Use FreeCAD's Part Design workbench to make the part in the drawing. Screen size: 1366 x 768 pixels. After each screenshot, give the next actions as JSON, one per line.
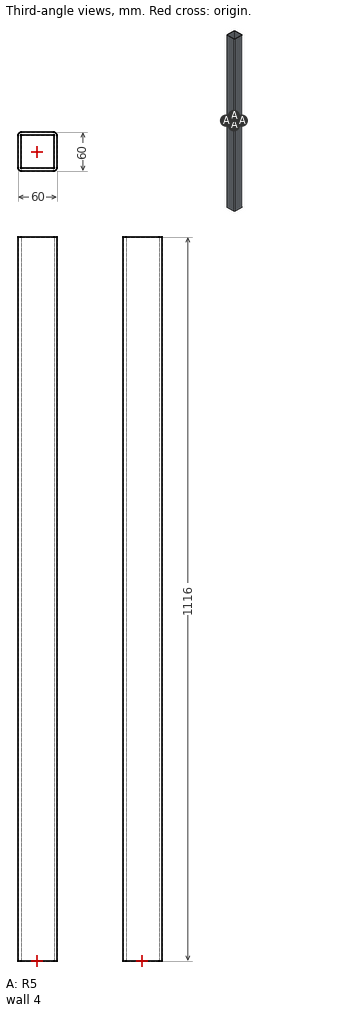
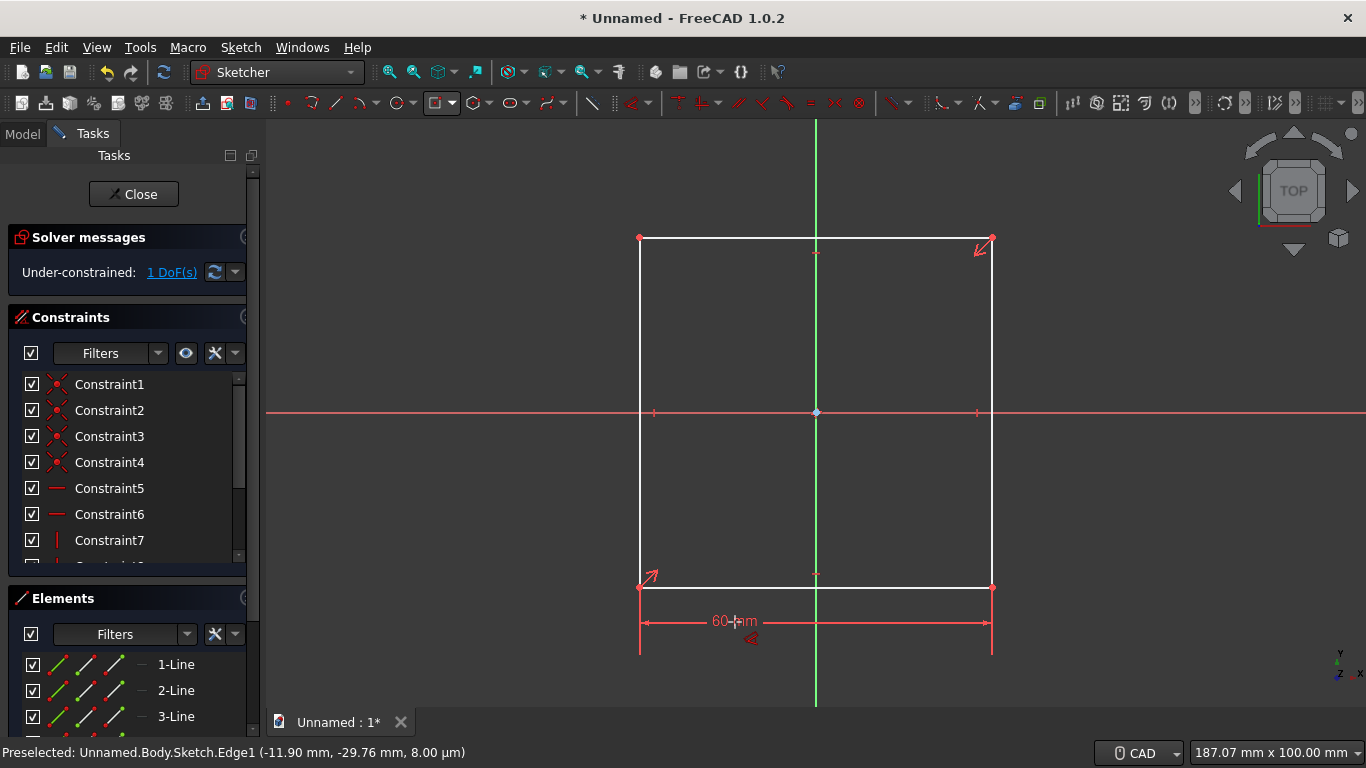
{"action": "left_click", "coordinate": [992, 483]}
{"action": "left_click", "coordinate": [1026, 333]}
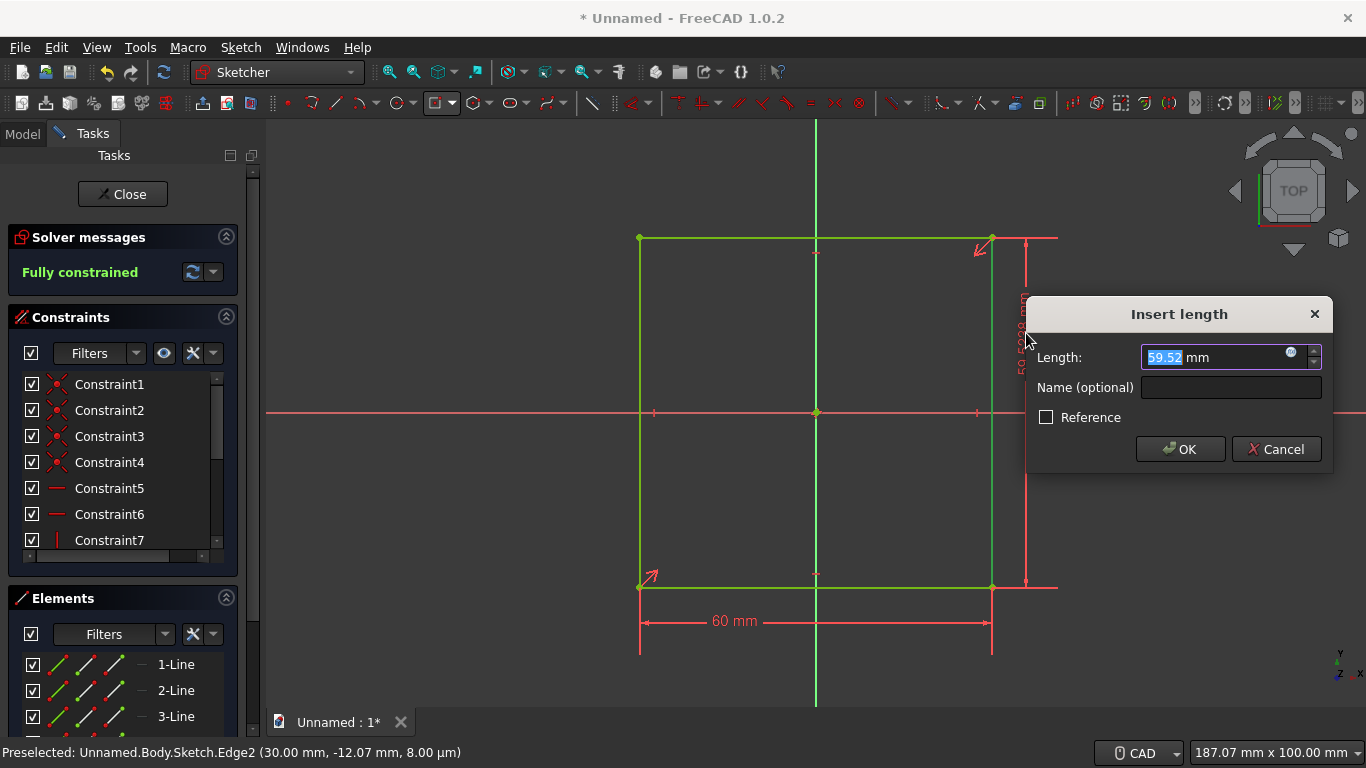
{"action": "type", "text": "60"}
{"action": "key", "text": "Return"}
{"action": "key", "text": "Escape"}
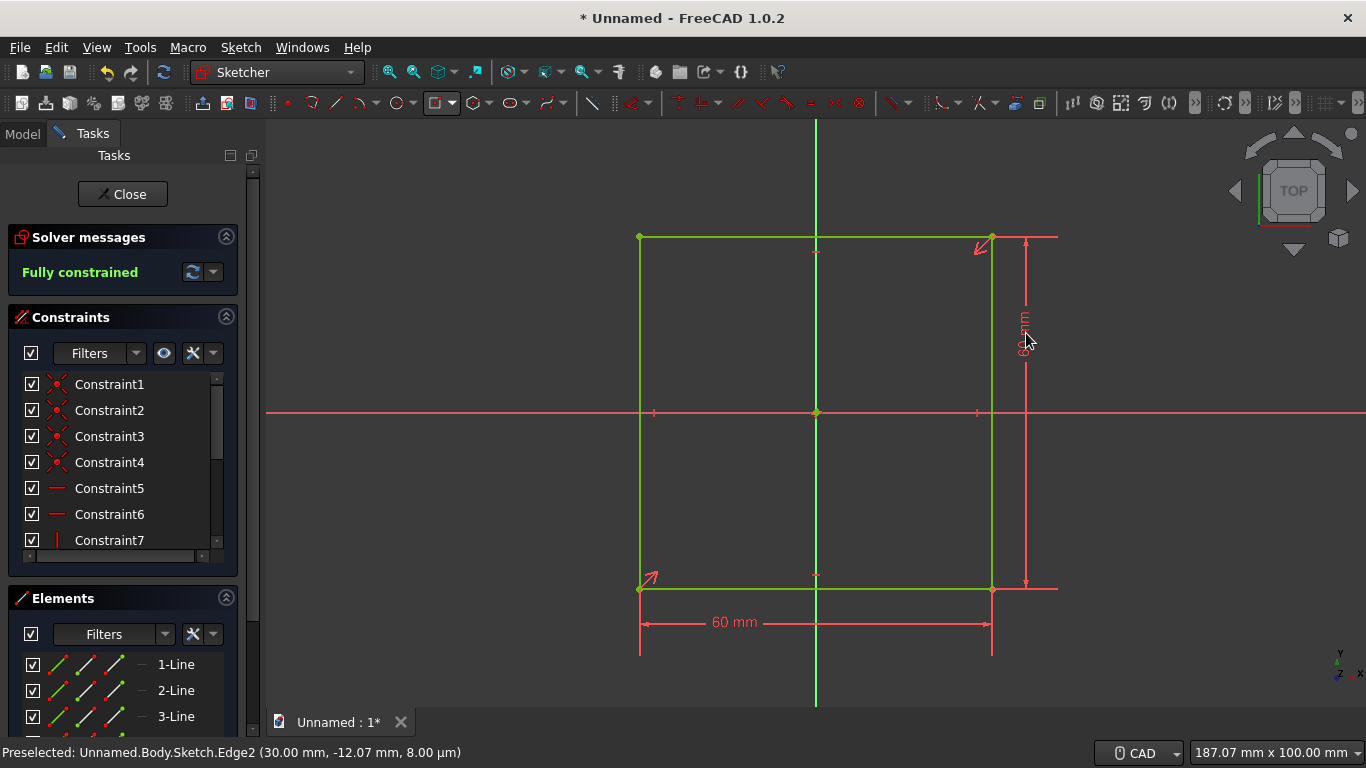
{"action": "left_click", "coordinate": [123, 194]}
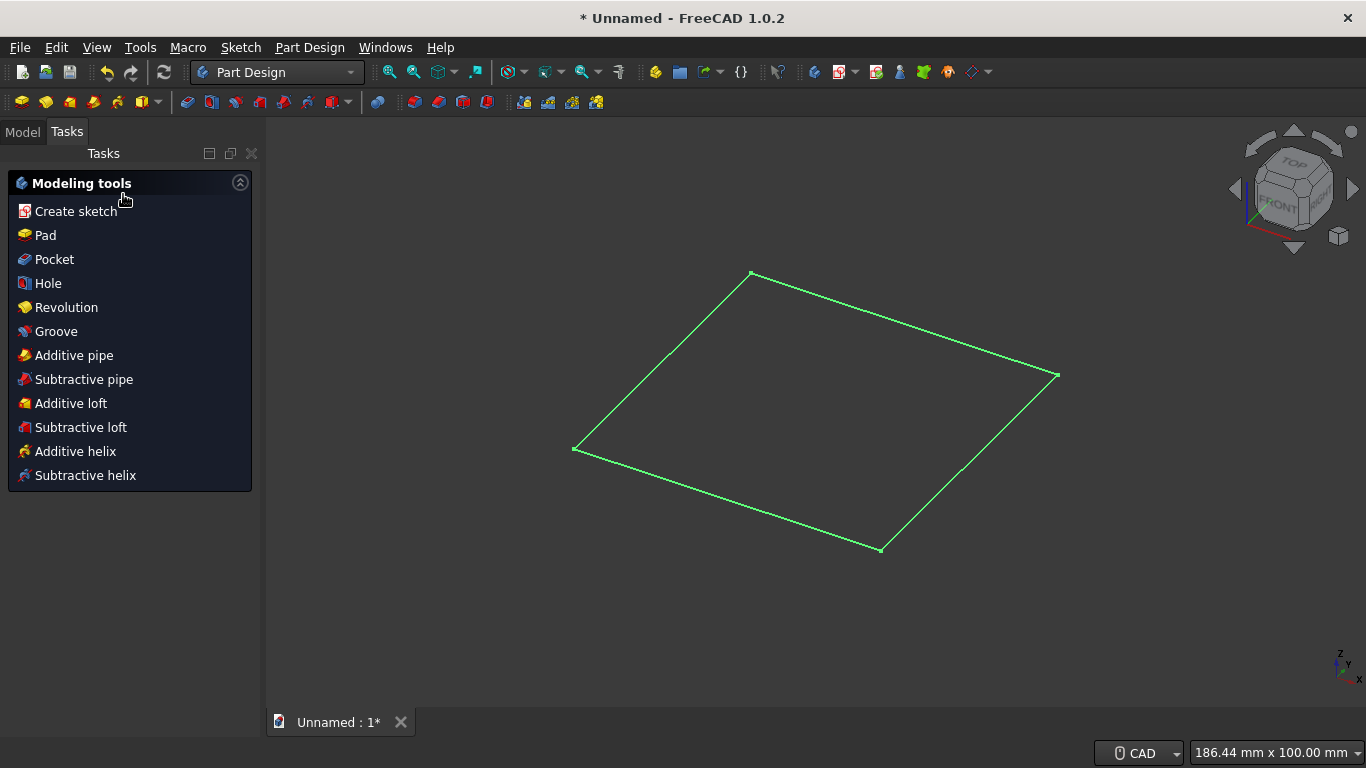
{"action": "left_click", "coordinate": [22, 102]}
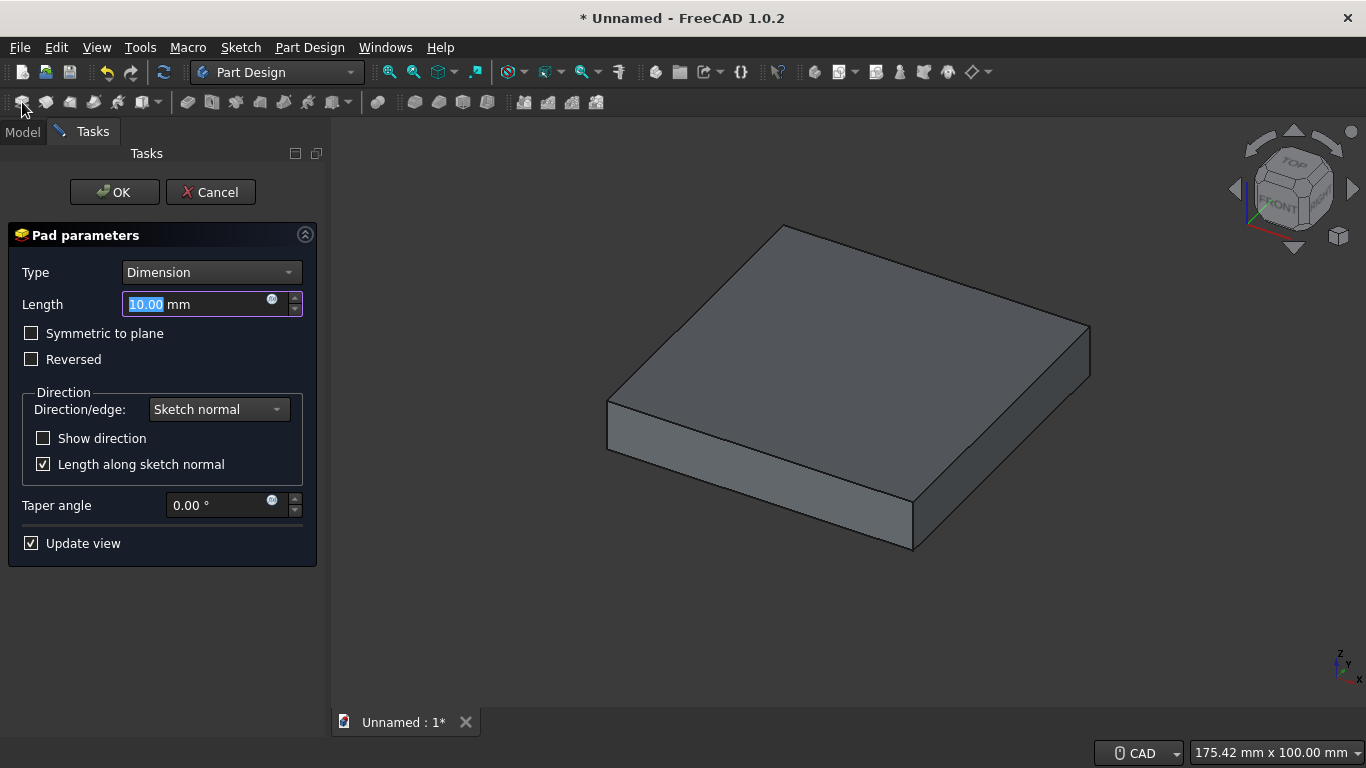
{"action": "type", "text": "1116"}
{"action": "key", "text": "Tab"}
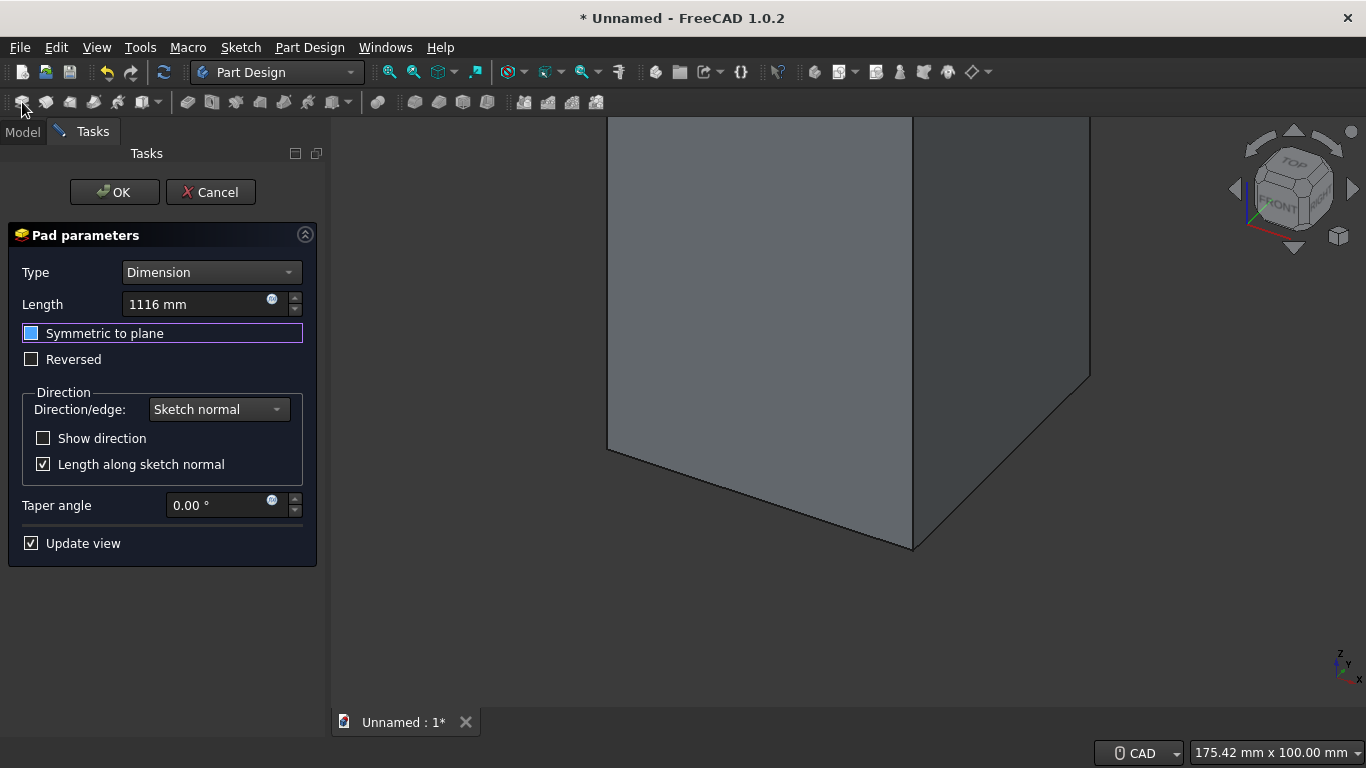
{"action": "left_click", "coordinate": [115, 192]}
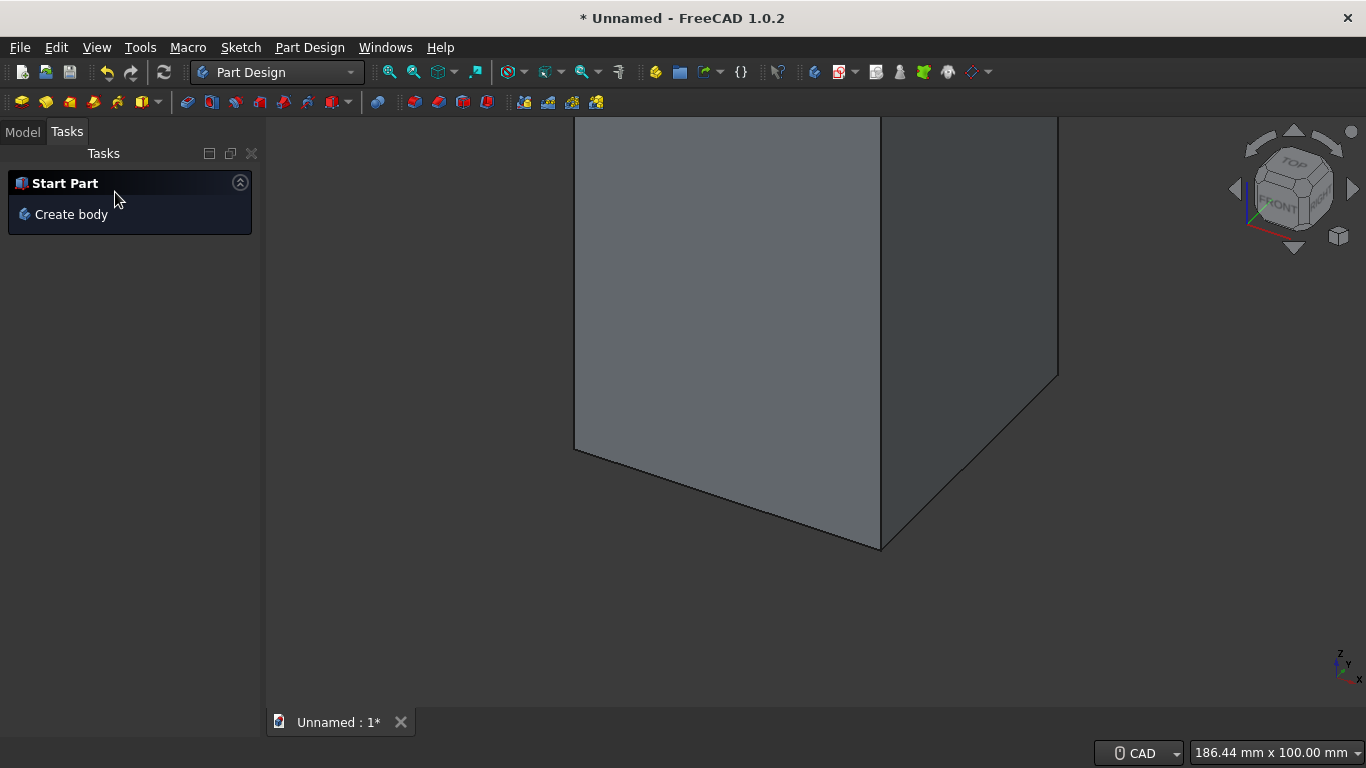
{"action": "left_click", "coordinate": [390, 72]}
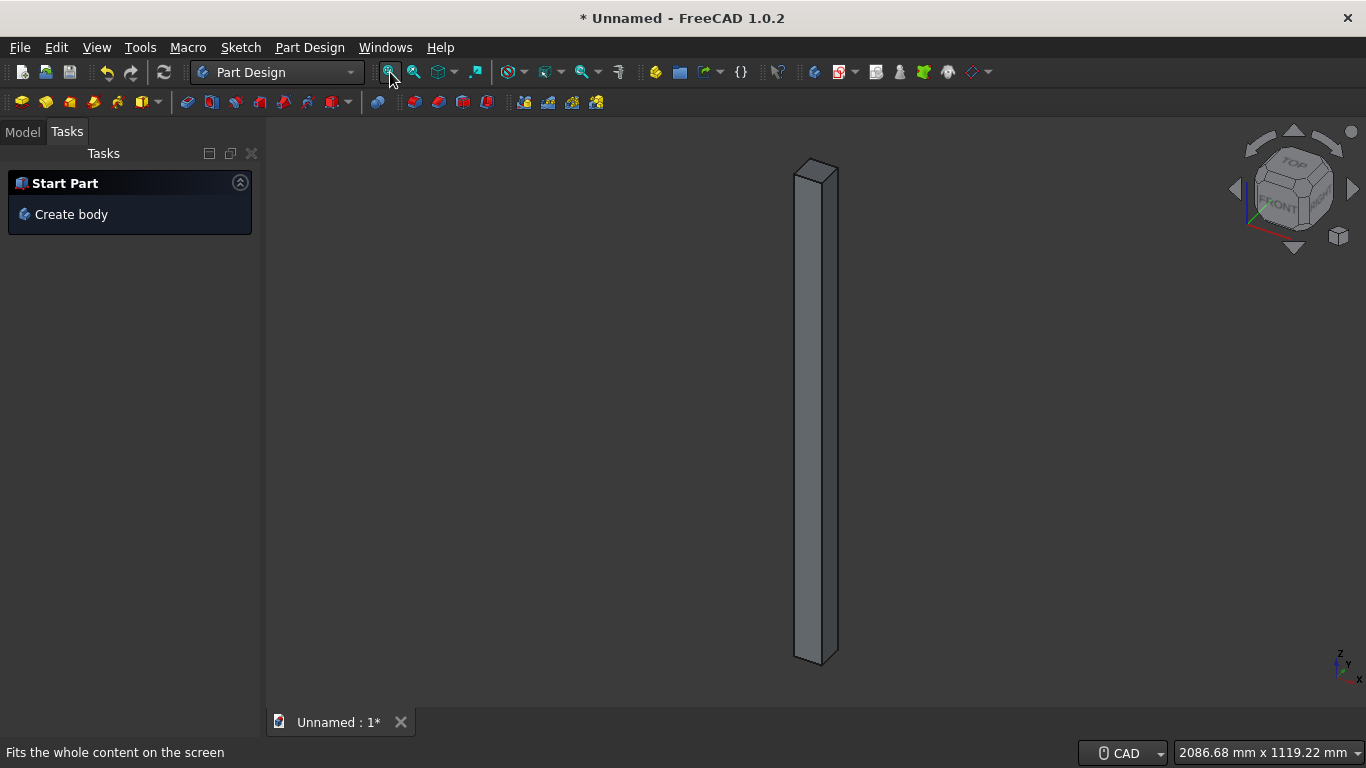
{"action": "left_click", "coordinate": [822, 423]}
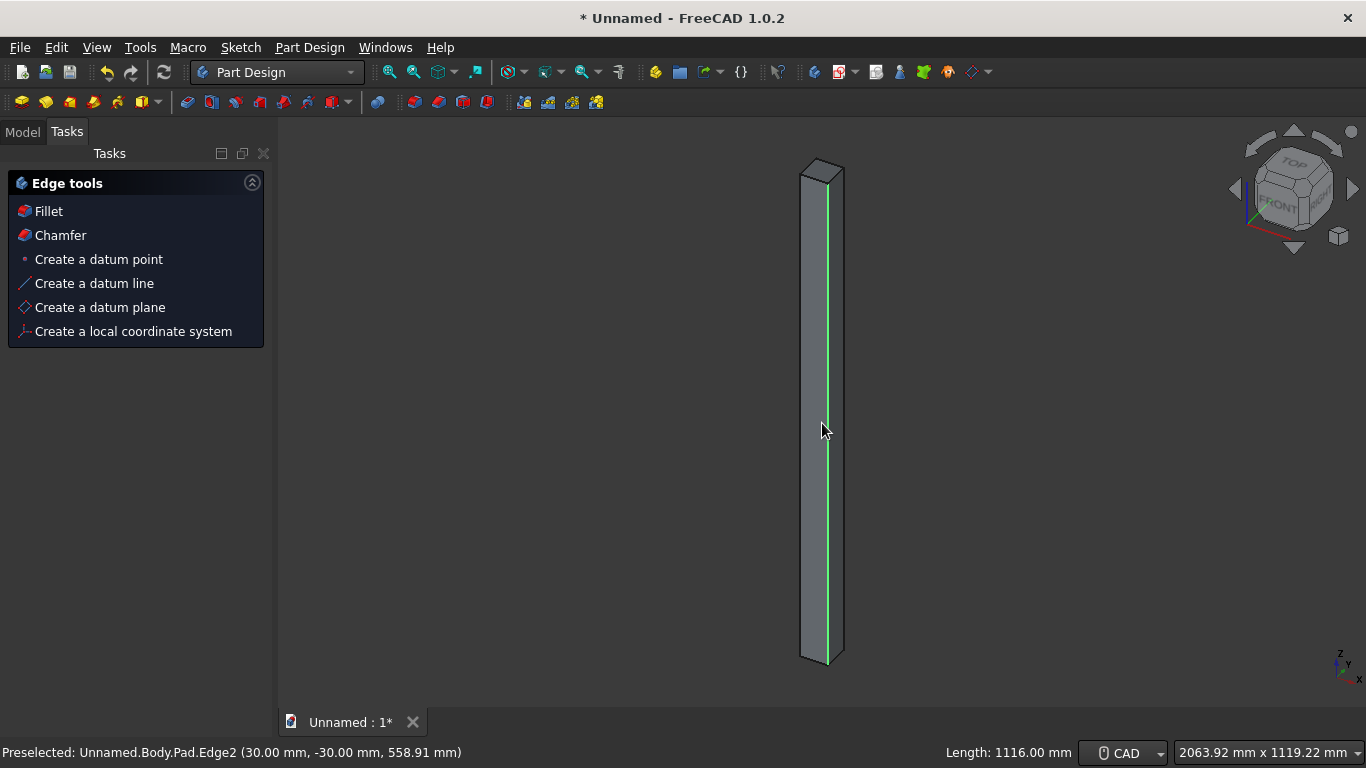
{"action": "key", "text": "0"}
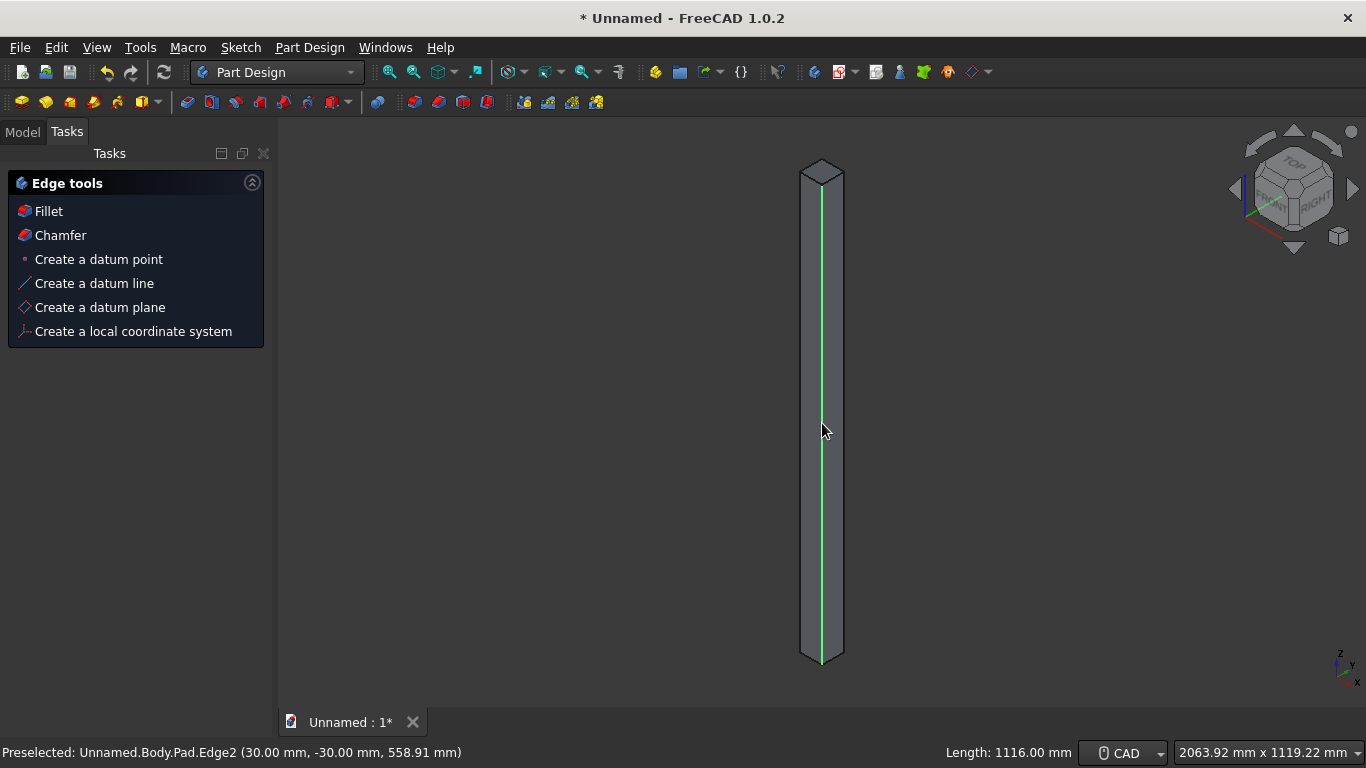
{"action": "key", "text": "2"}